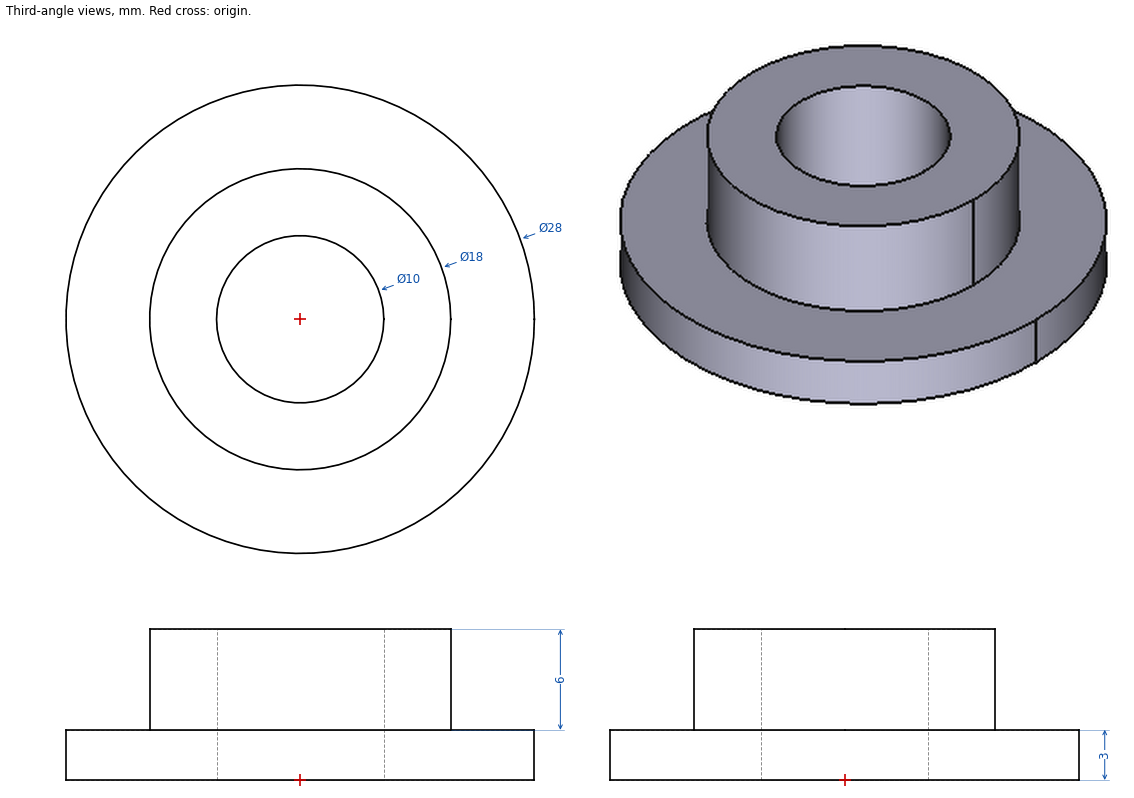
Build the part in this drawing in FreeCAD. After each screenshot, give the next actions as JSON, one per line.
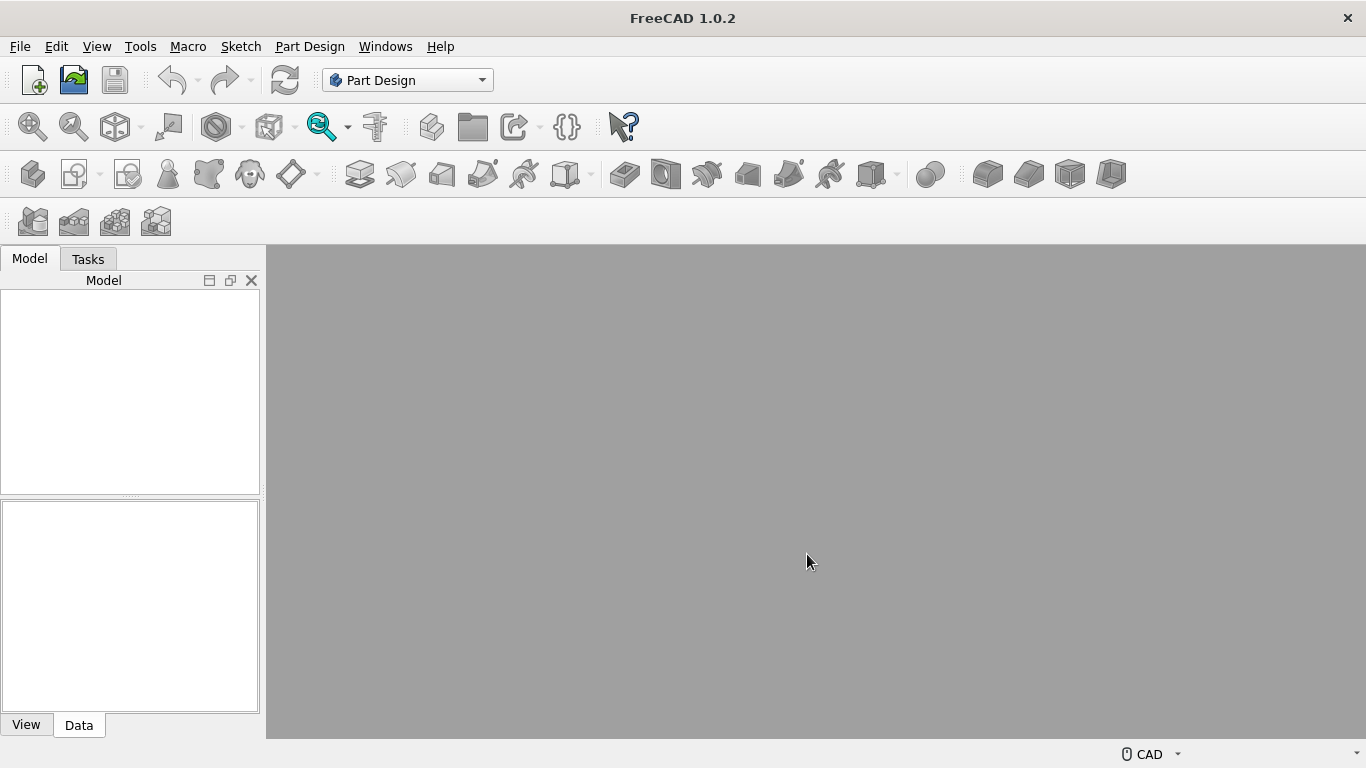
{"action": "key", "text": "ctrl+n"}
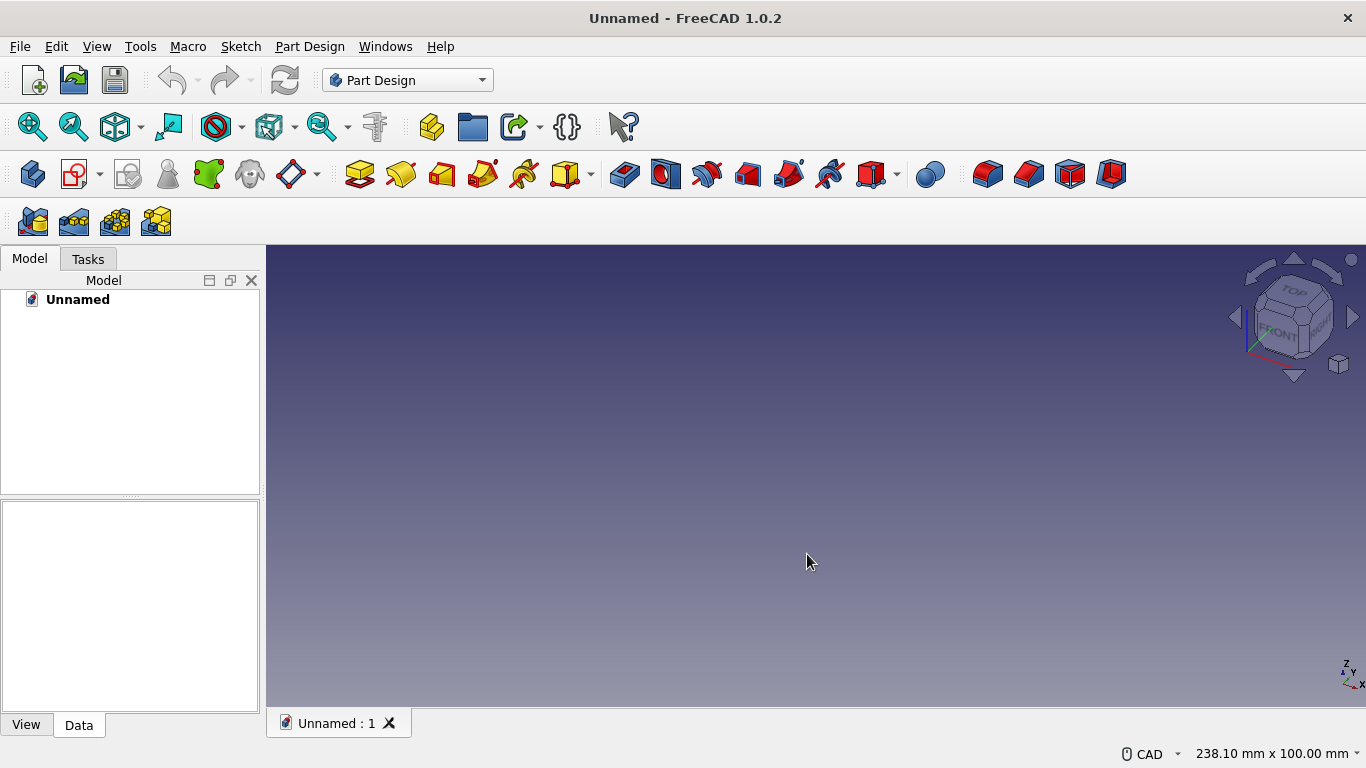
{"action": "left_click", "coordinate": [74, 174]}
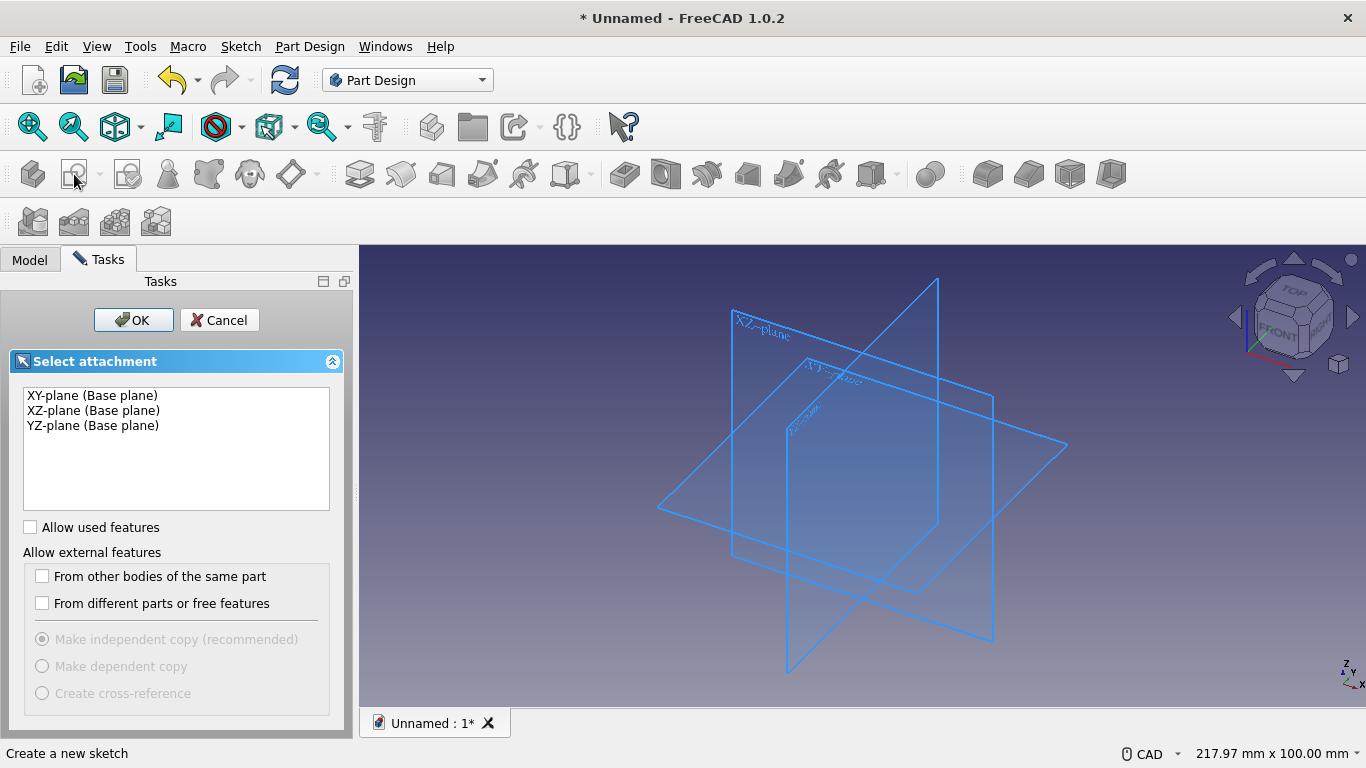
{"action": "left_click", "coordinate": [84, 396]}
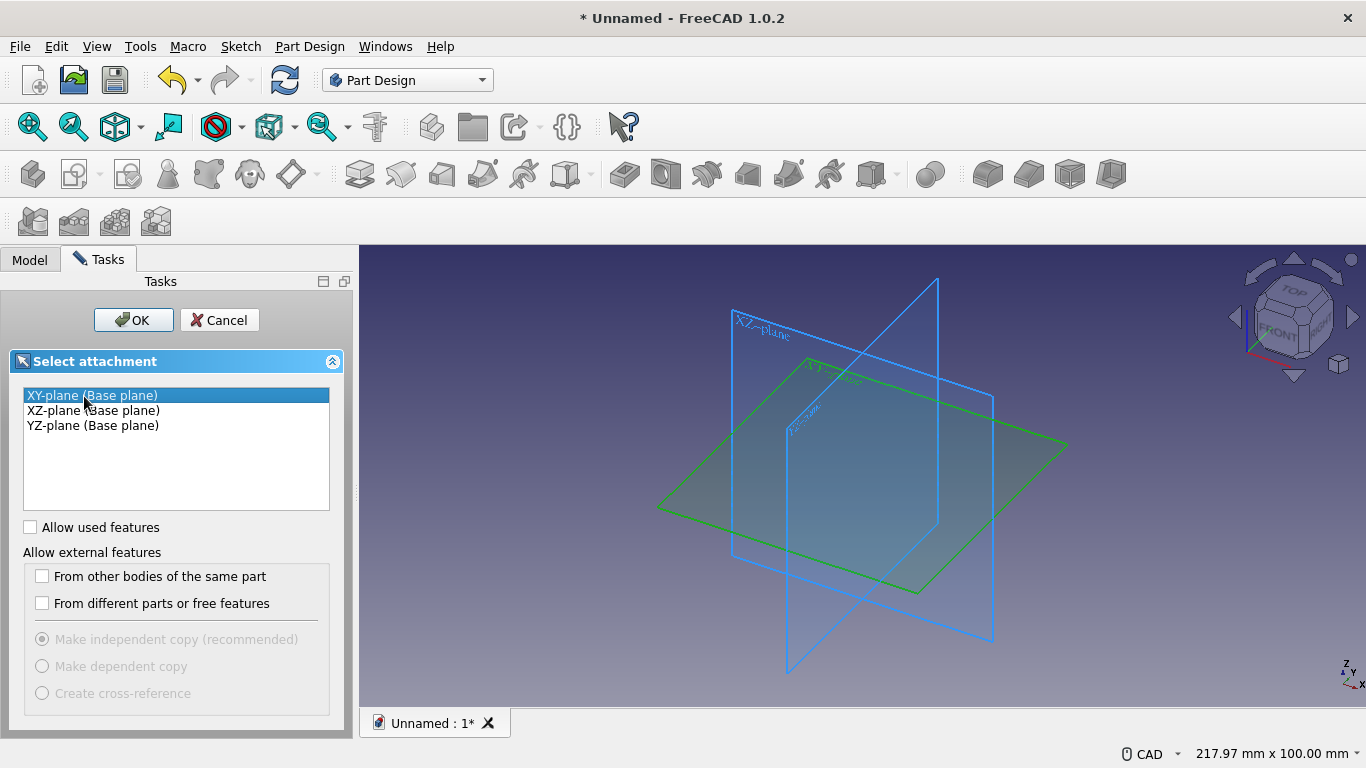
{"action": "left_click", "coordinate": [134, 320]}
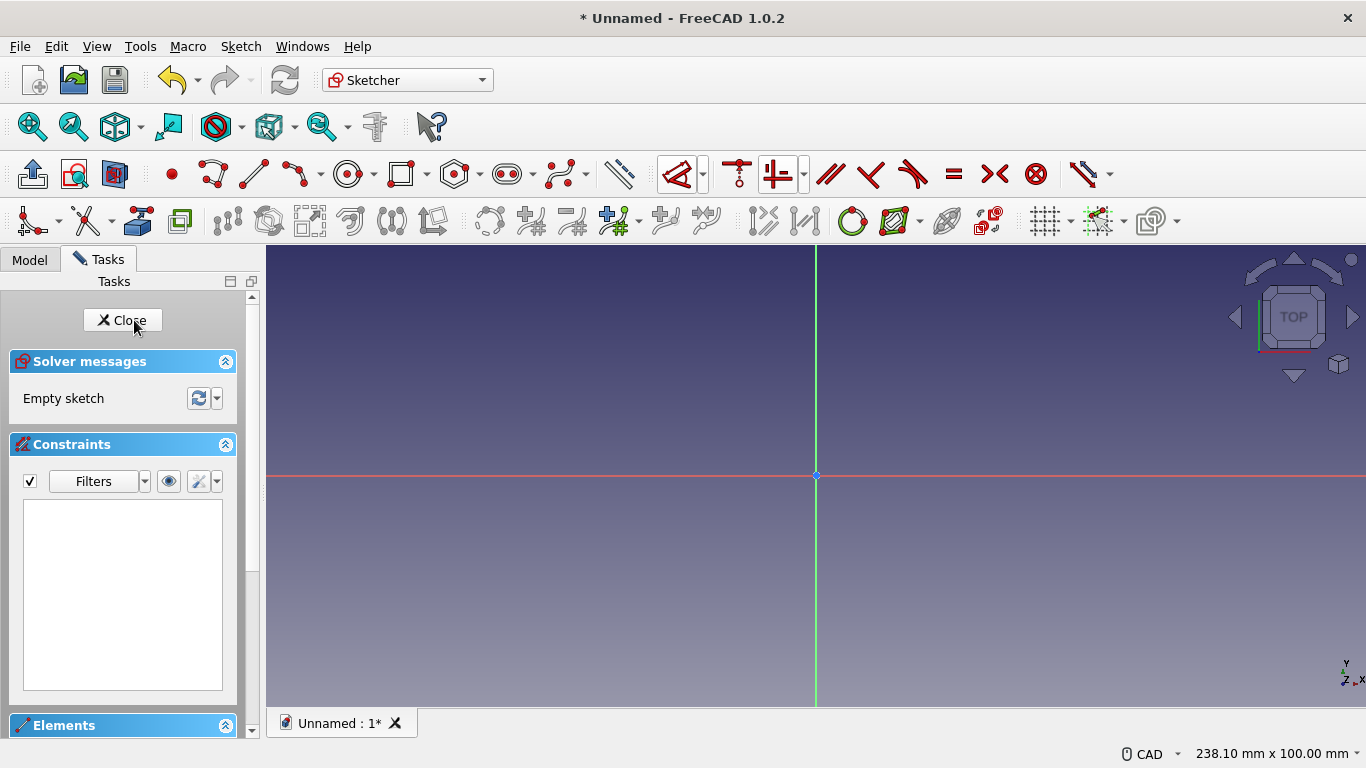
{"action": "scroll", "coordinate": [872, 476], "scroll_direction": "up", "scroll_amount": 4}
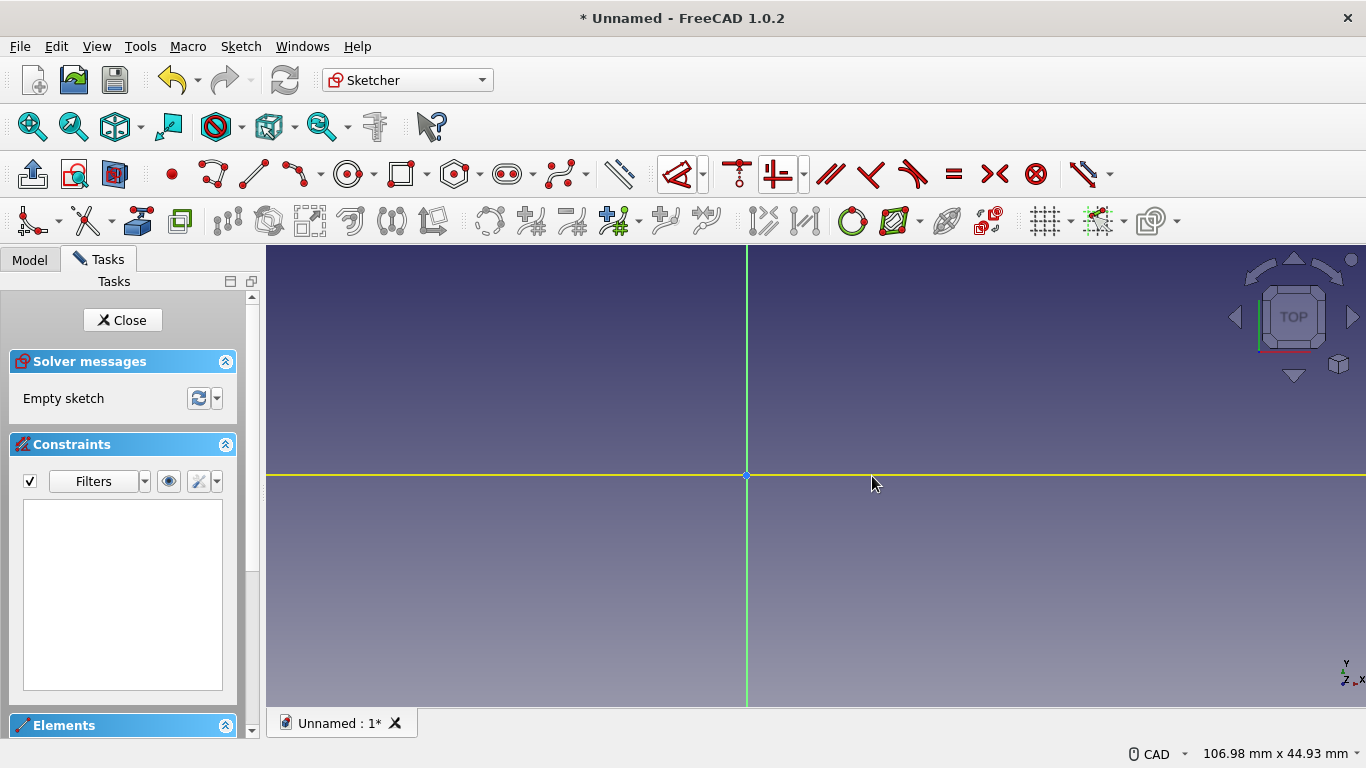
{"action": "left_click", "coordinate": [348, 174]}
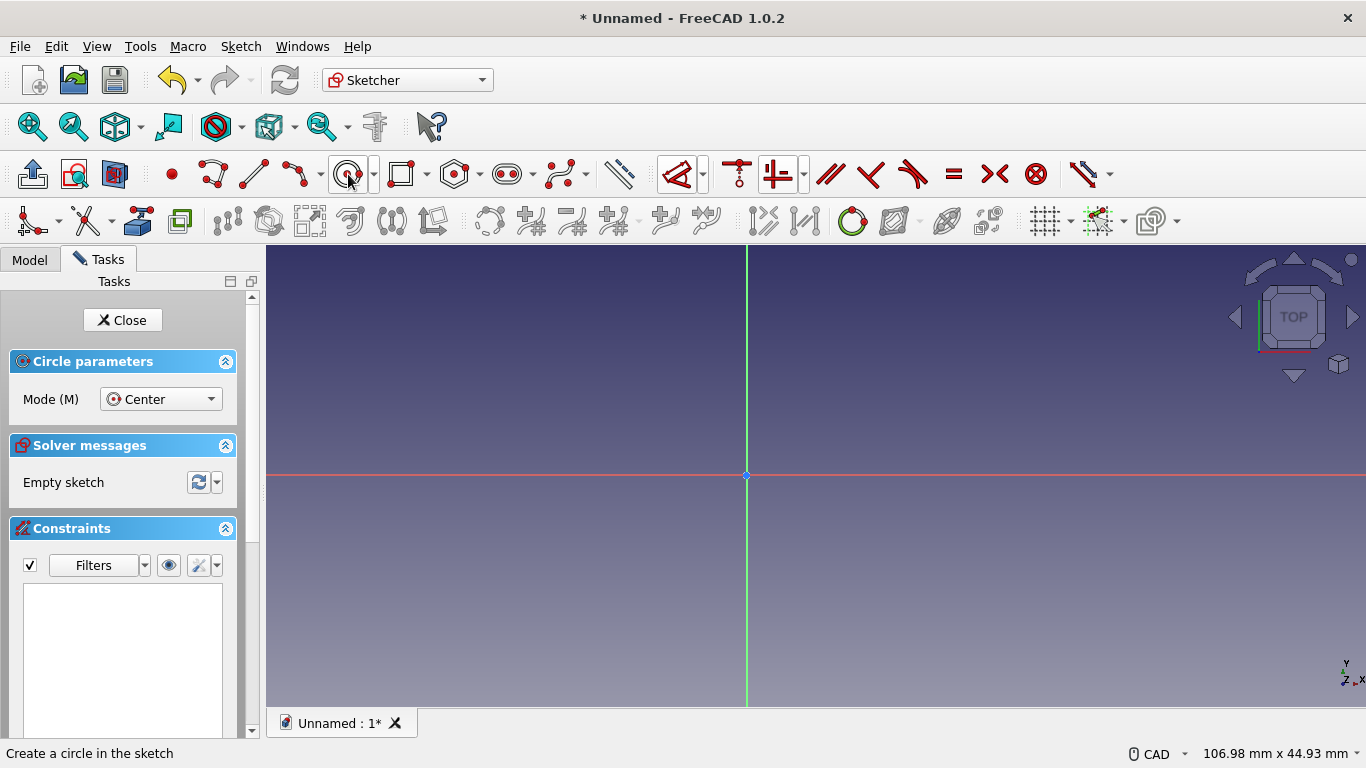
{"action": "left_click", "coordinate": [747, 475]}
{"action": "left_click", "coordinate": [848, 374]}
{"action": "key", "text": "Escape"}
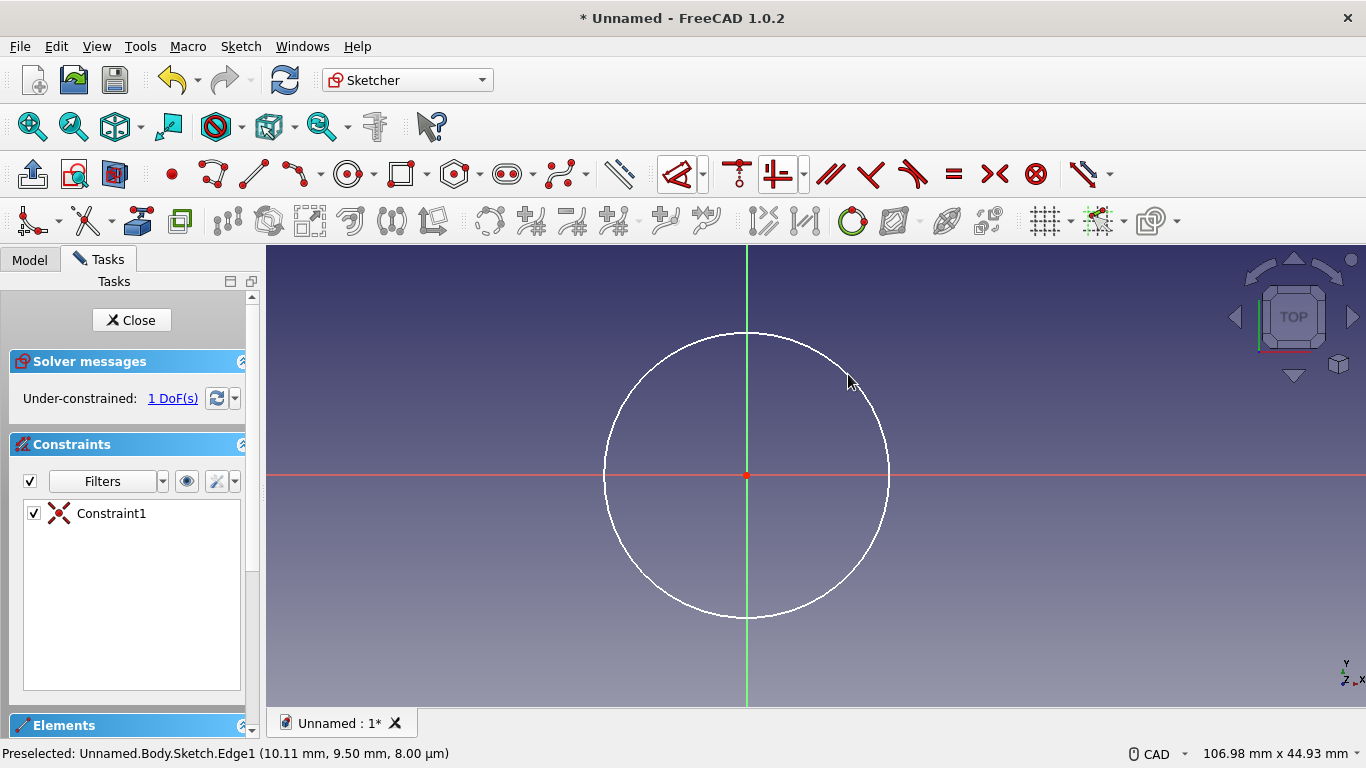
{"action": "left_click", "coordinate": [847, 374]}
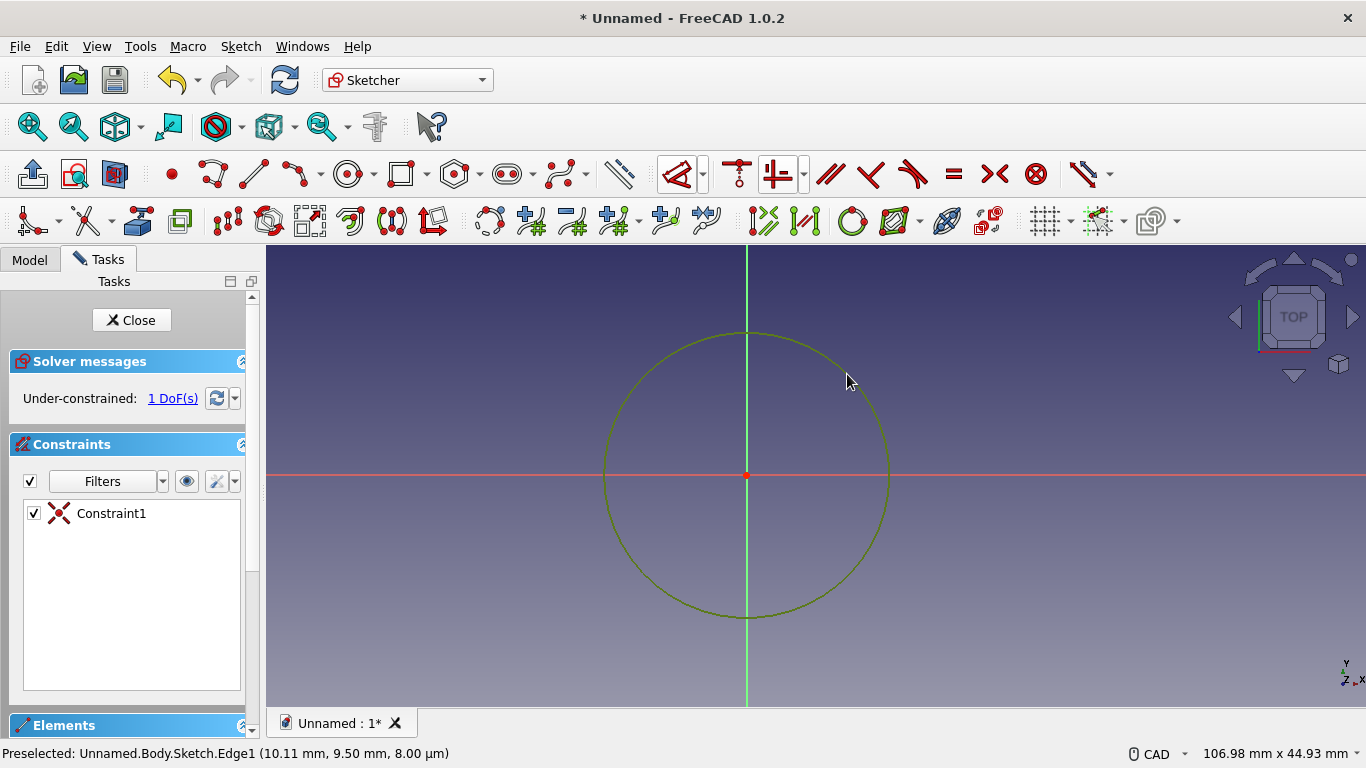
{"action": "key", "text": "k o"}